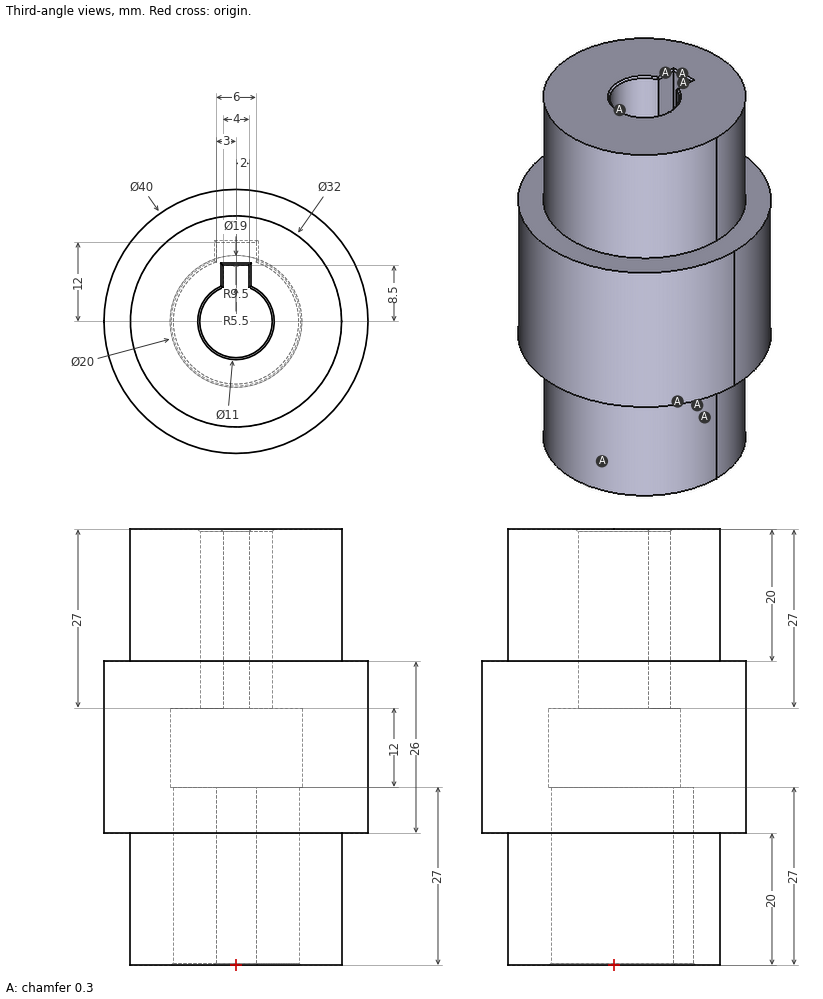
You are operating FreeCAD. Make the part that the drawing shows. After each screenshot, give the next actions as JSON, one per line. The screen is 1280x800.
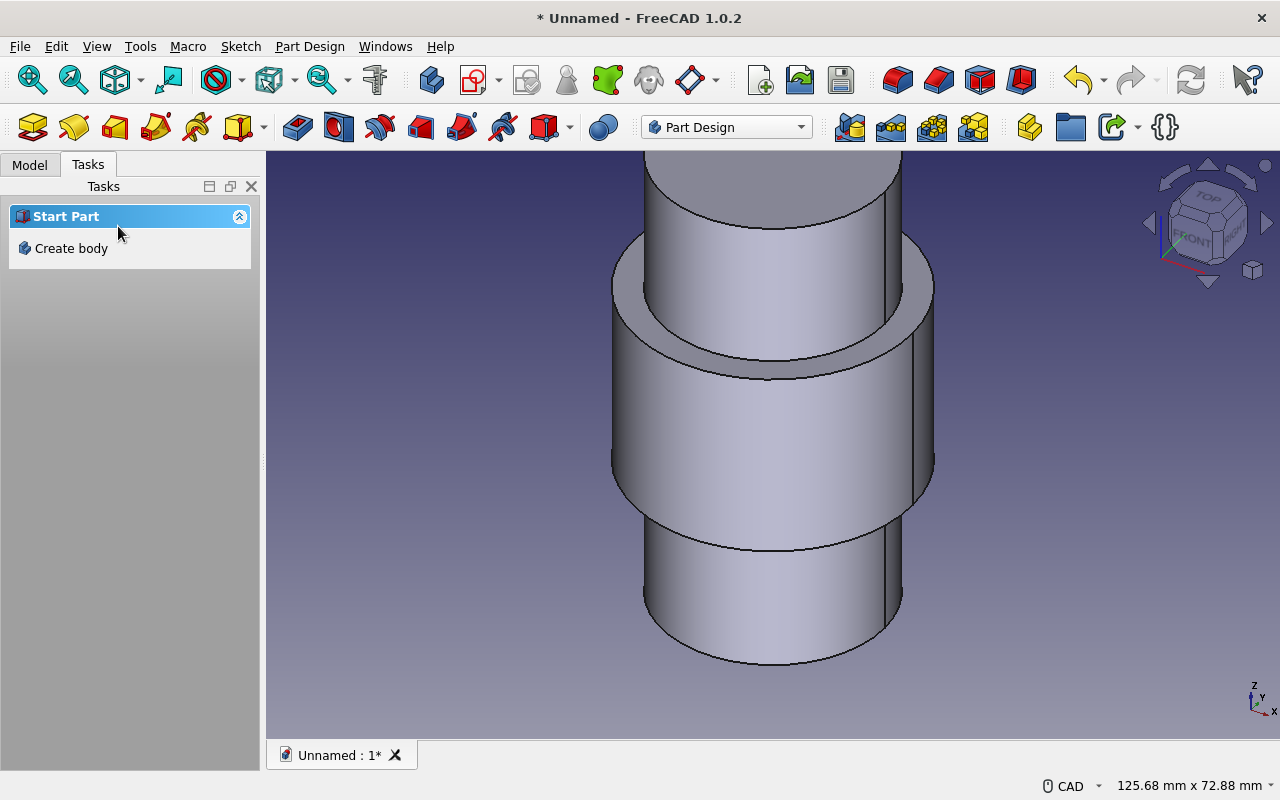
{"action": "left_click", "coordinate": [33, 80]}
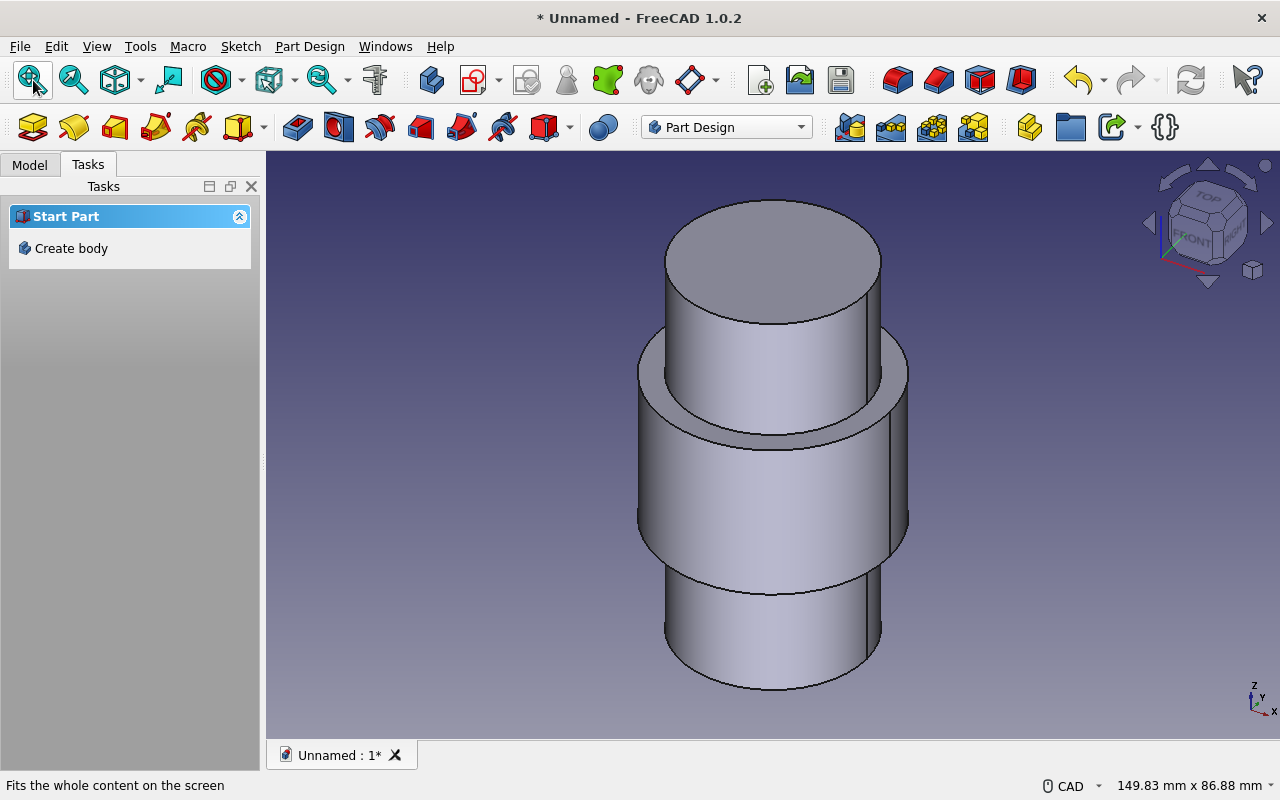
{"action": "left_click", "coordinate": [472, 80]}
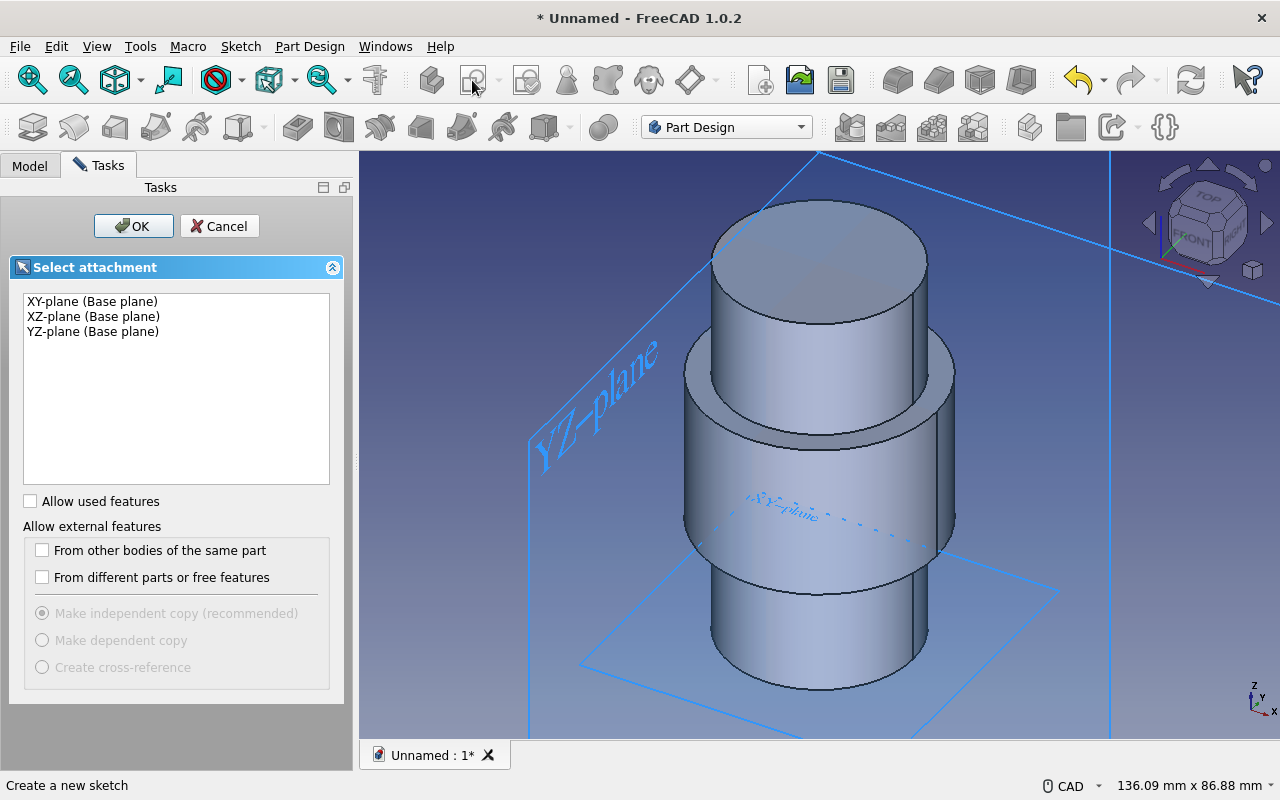
{"action": "left_click", "coordinate": [84, 302]}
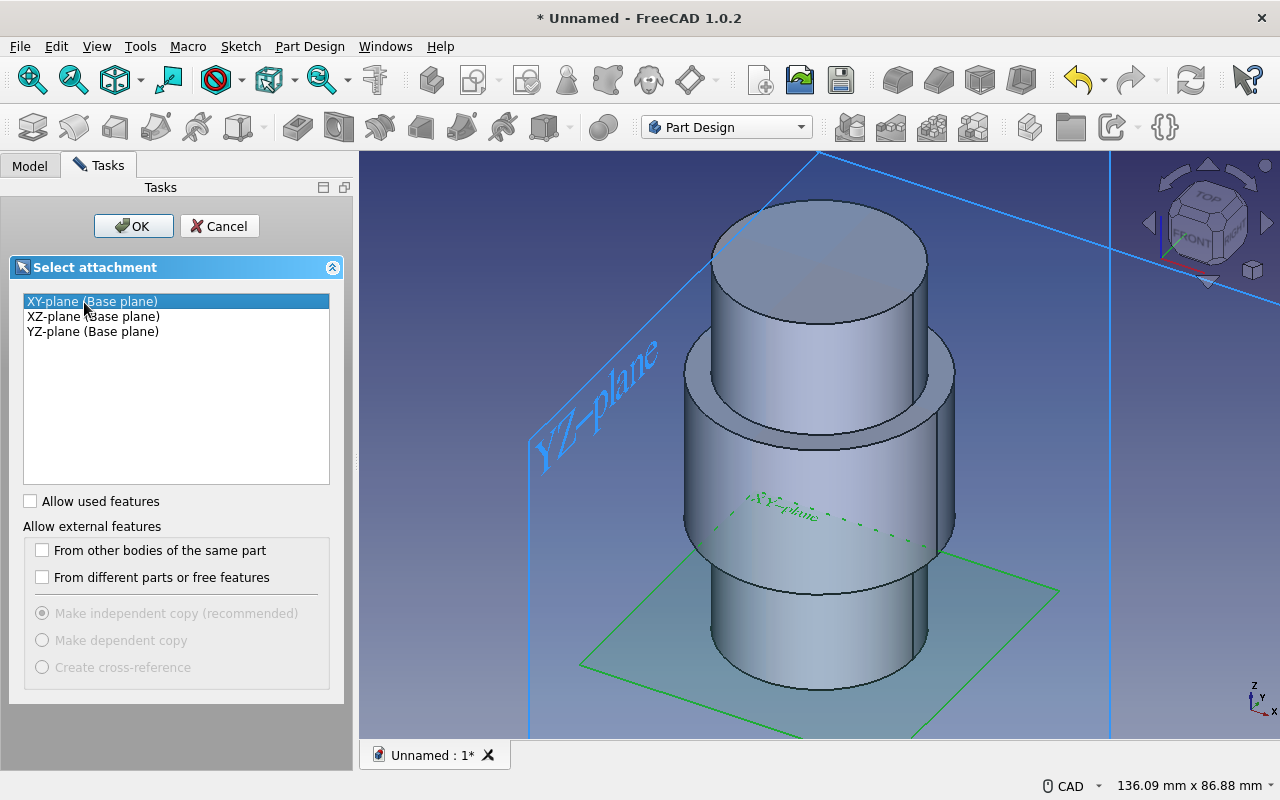
{"action": "left_click", "coordinate": [134, 226]}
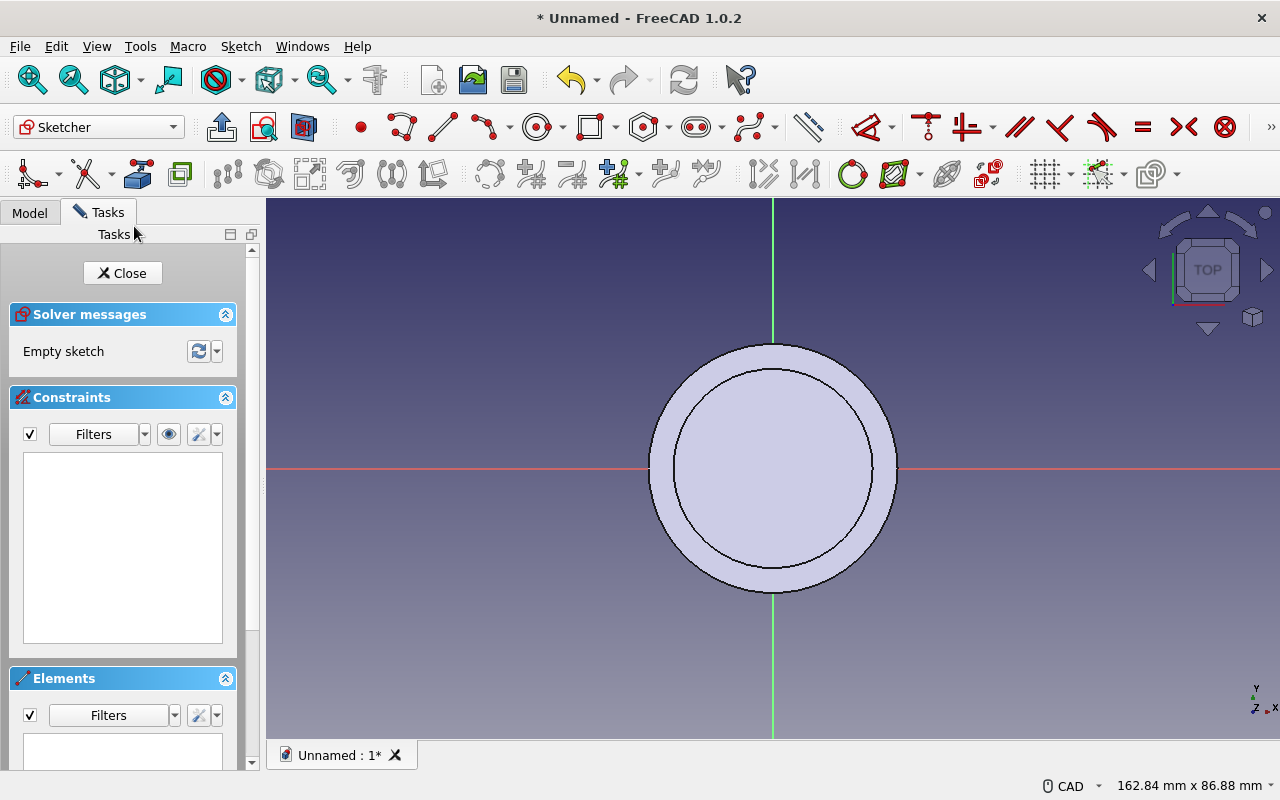
{"action": "left_click", "coordinate": [304, 128]}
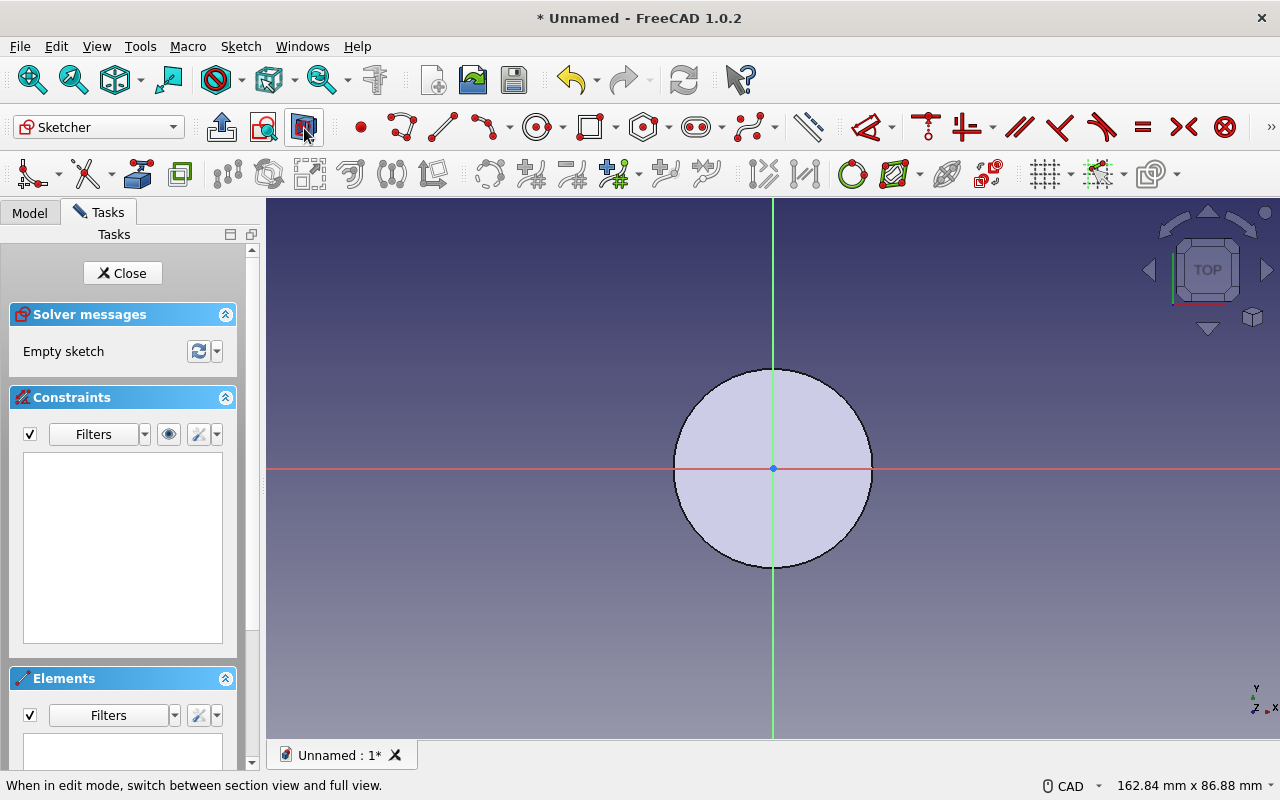
{"action": "scroll", "coordinate": [813, 468], "scroll_direction": "up", "scroll_amount": 5}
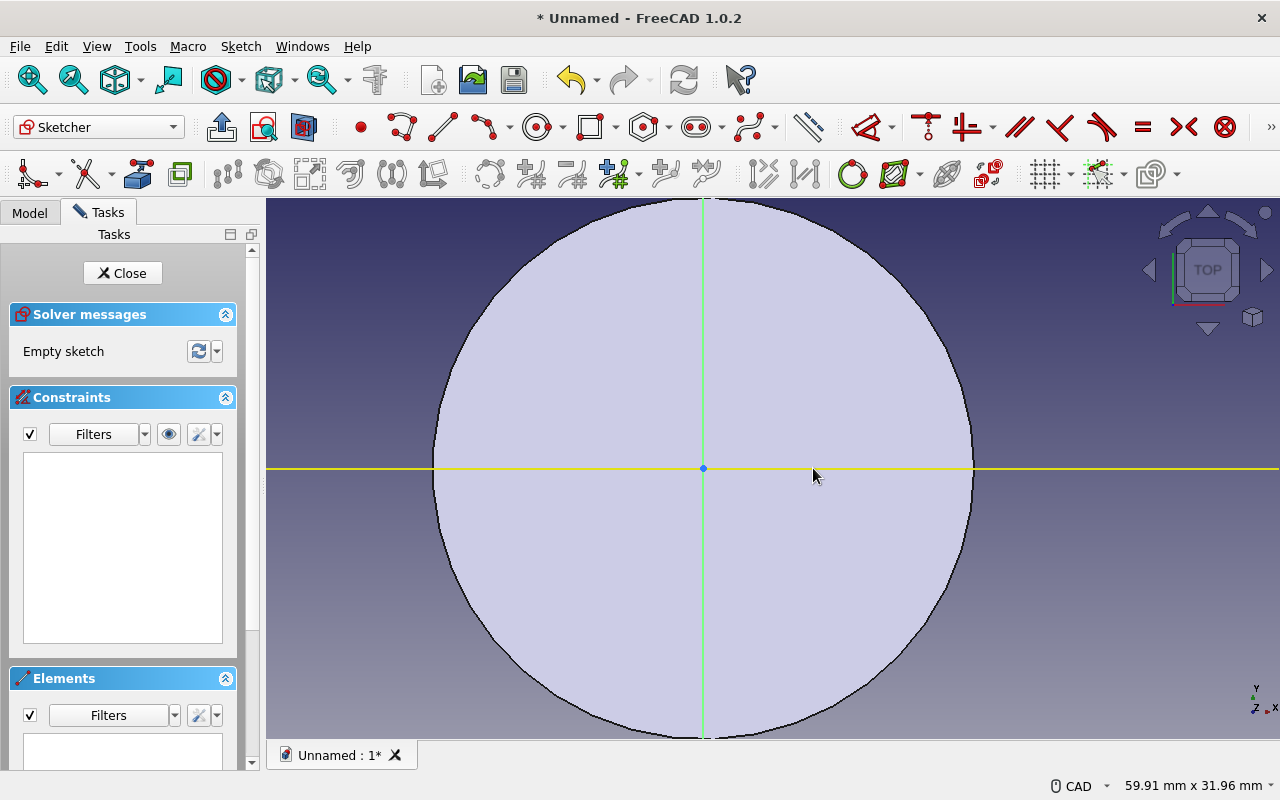
{"action": "left_click", "coordinate": [536, 128]}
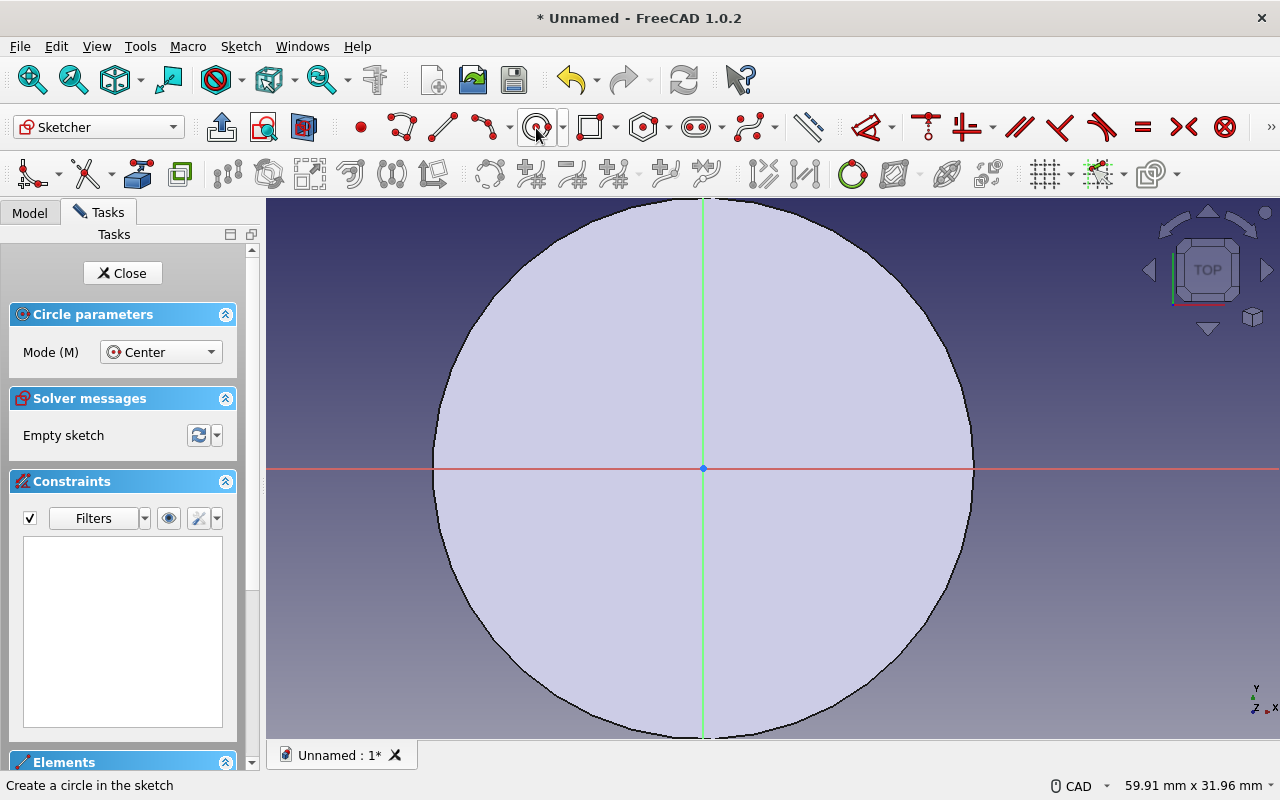
{"action": "left_click", "coordinate": [703, 468]}
{"action": "left_click", "coordinate": [817, 355]}
{"action": "key", "text": "Escape"}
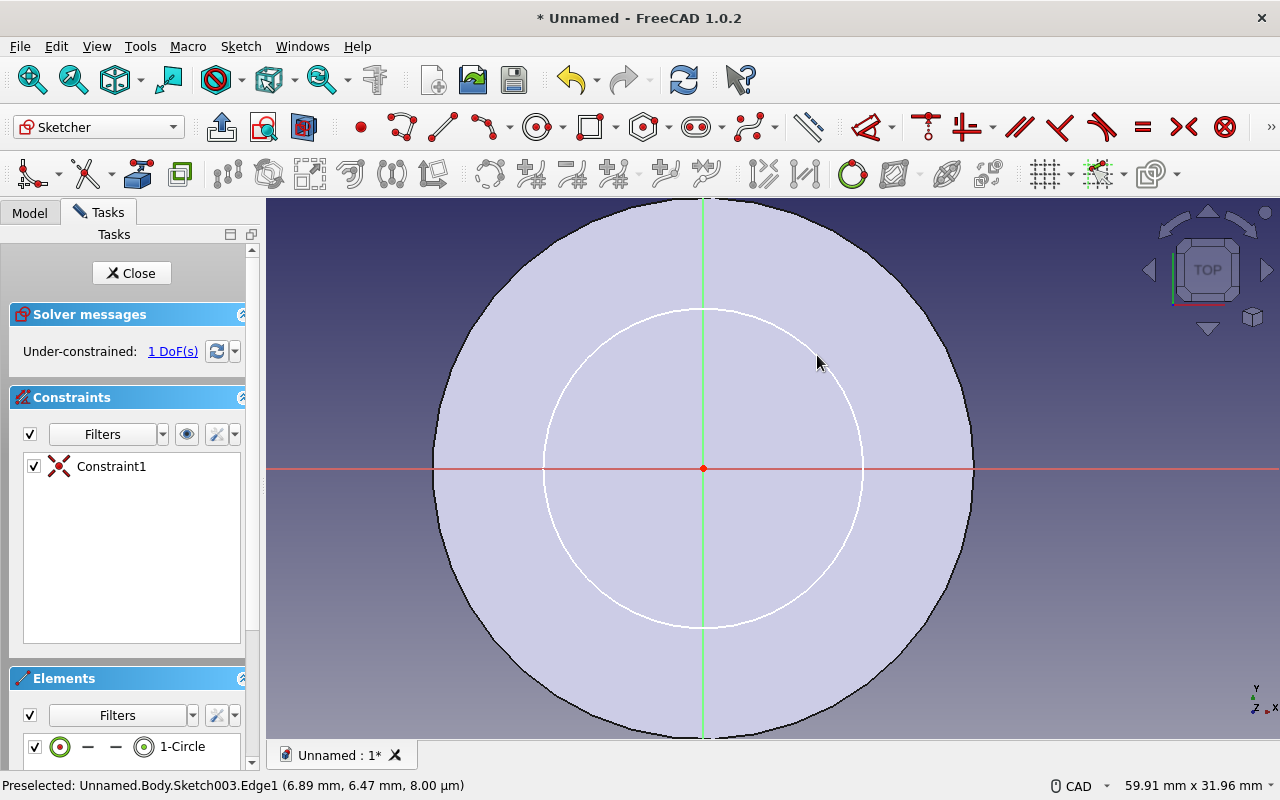
{"action": "left_click", "coordinate": [866, 128]}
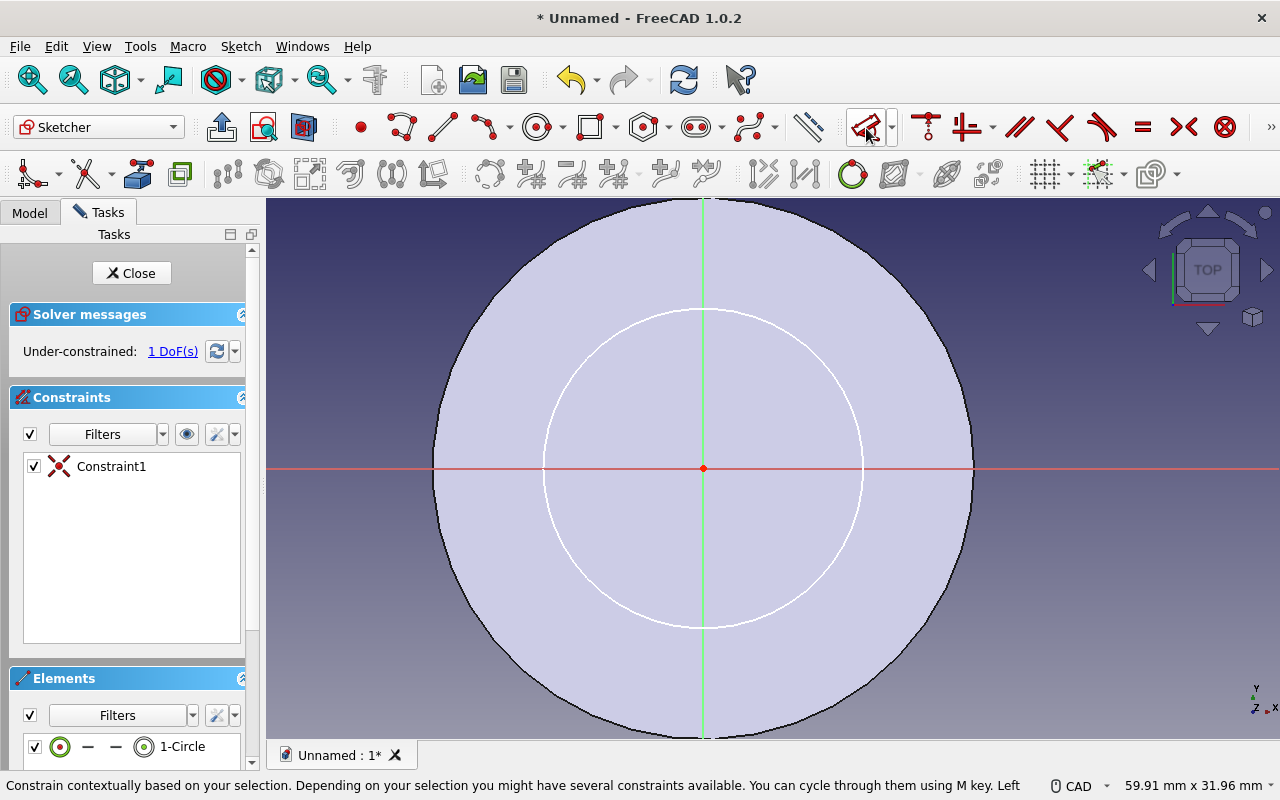
{"action": "left_click", "coordinate": [816, 355]}
{"action": "left_click", "coordinate": [839, 332]}